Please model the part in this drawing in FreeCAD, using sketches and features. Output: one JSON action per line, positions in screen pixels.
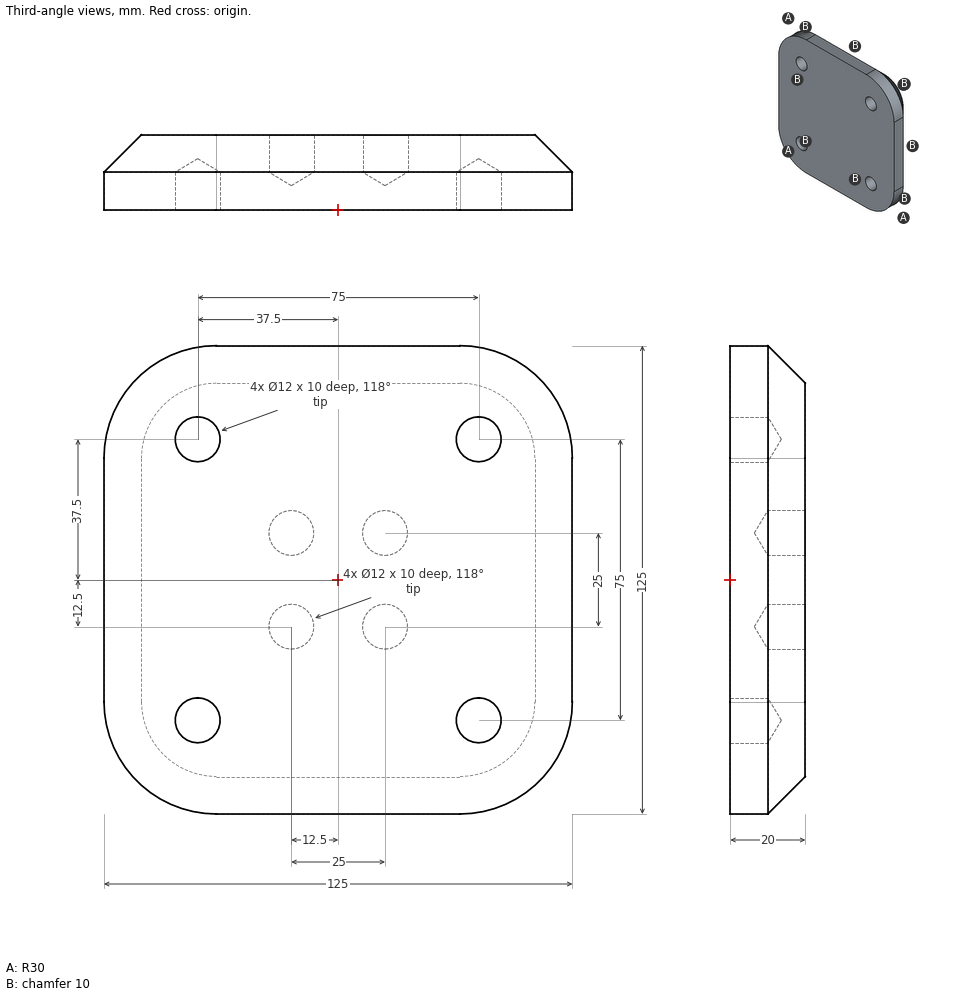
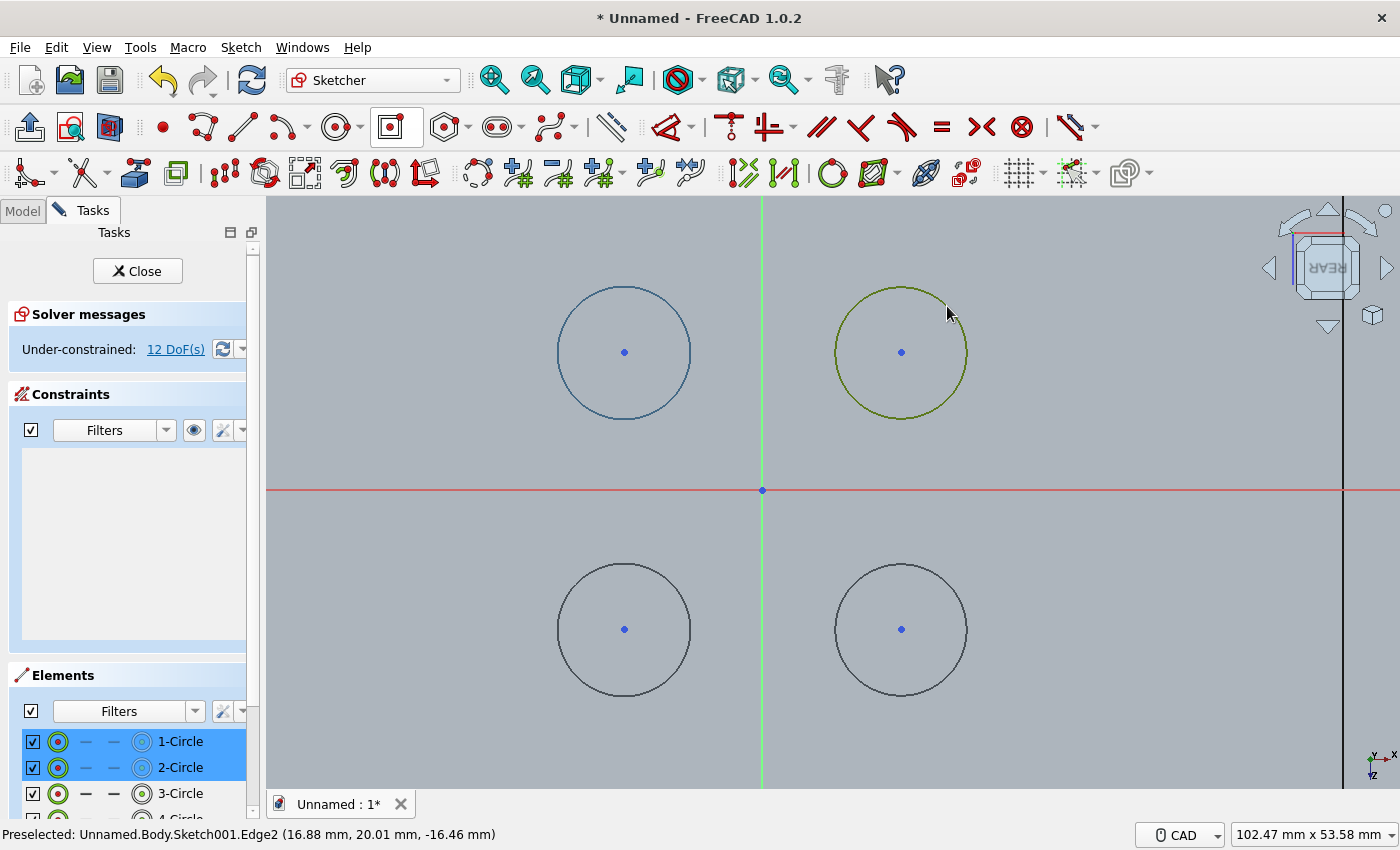
{"action": "left_click", "coordinate": [947, 583]}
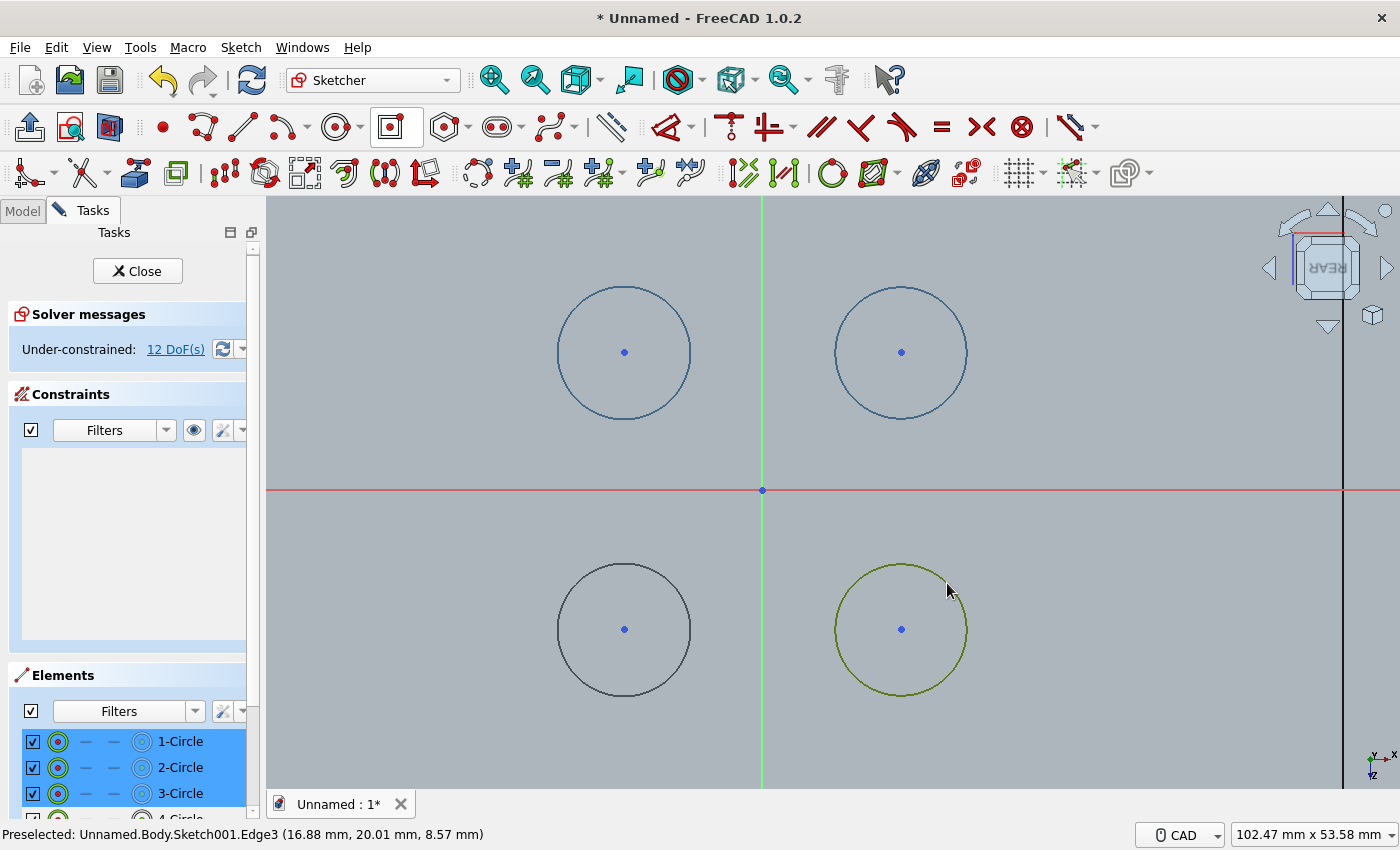
{"action": "left_click", "coordinate": [671, 583]}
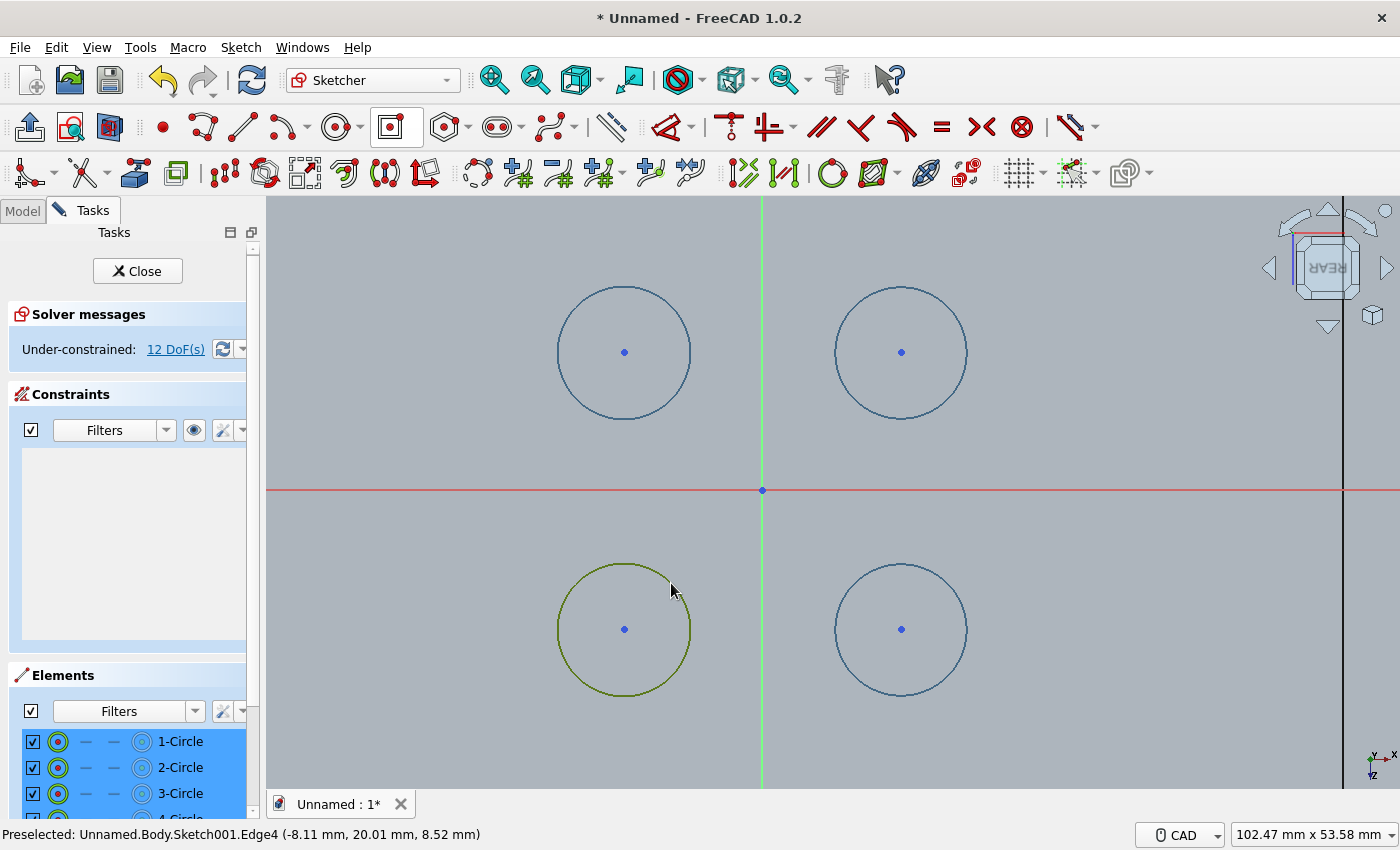
{"action": "left_click", "coordinate": [942, 128]}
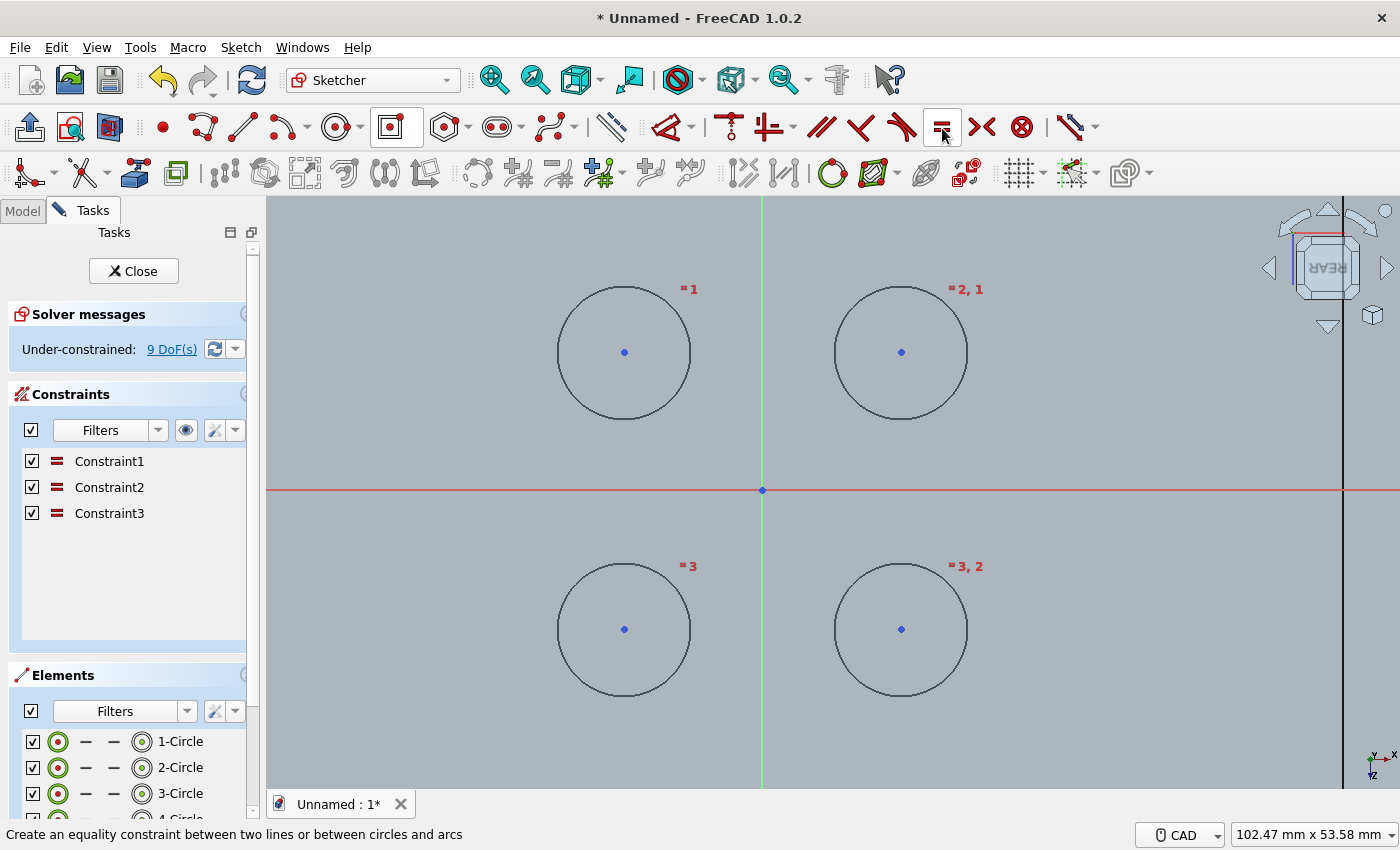
{"action": "left_click", "coordinate": [624, 353]}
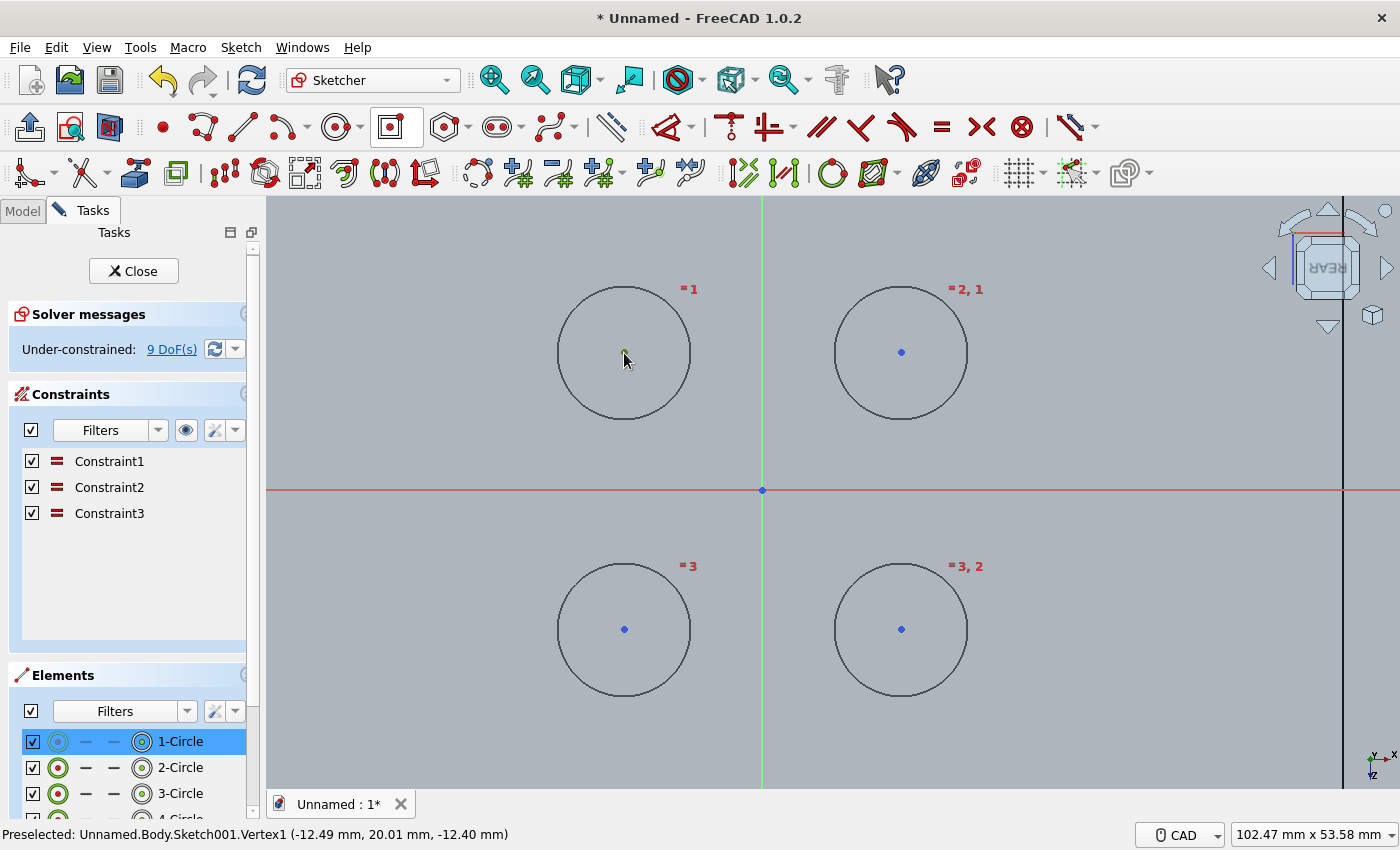
{"action": "left_click", "coordinate": [901, 353]}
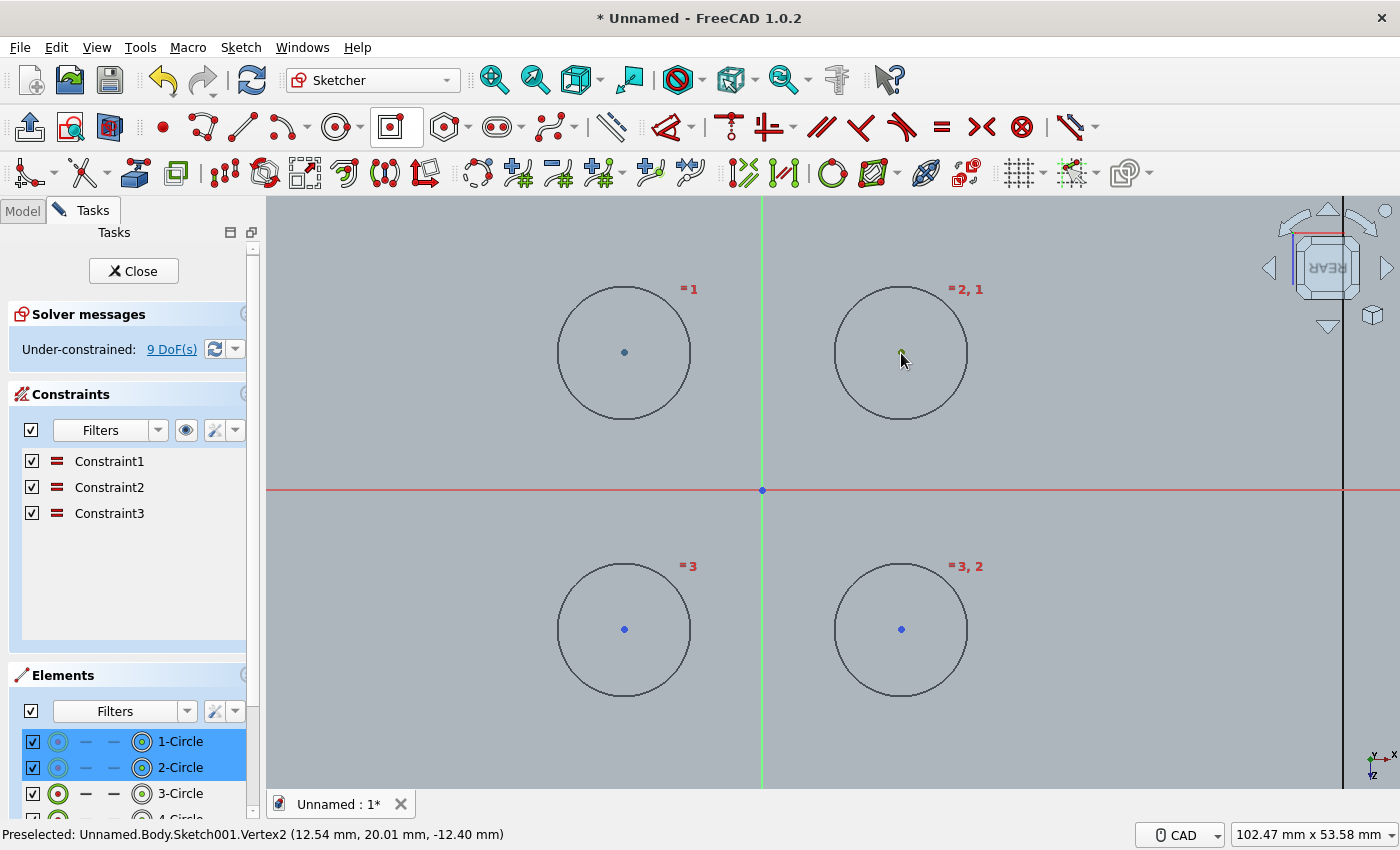
{"action": "key", "text": "h"}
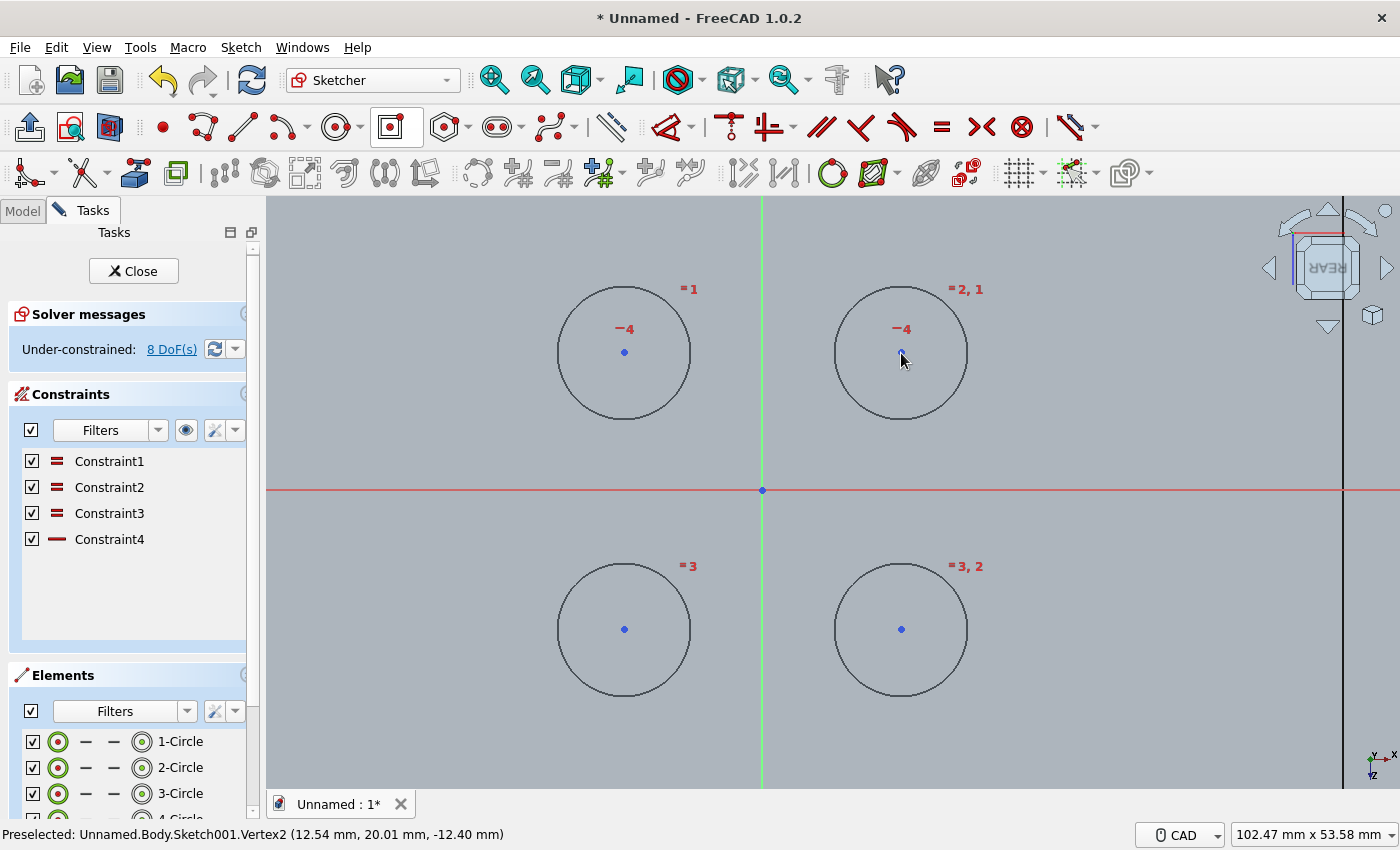
{"action": "left_click", "coordinate": [901, 353]}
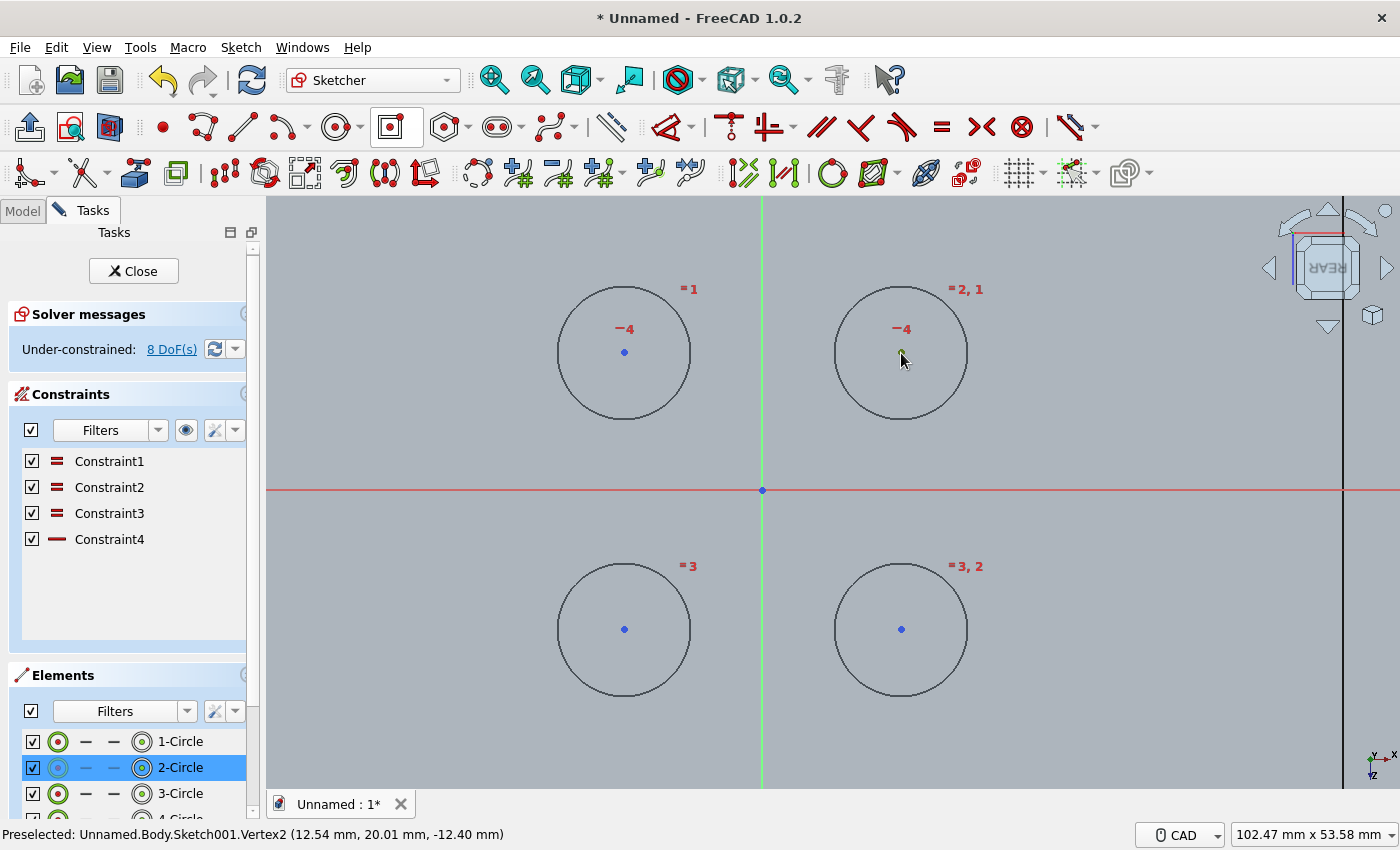
{"action": "left_click", "coordinate": [901, 630]}